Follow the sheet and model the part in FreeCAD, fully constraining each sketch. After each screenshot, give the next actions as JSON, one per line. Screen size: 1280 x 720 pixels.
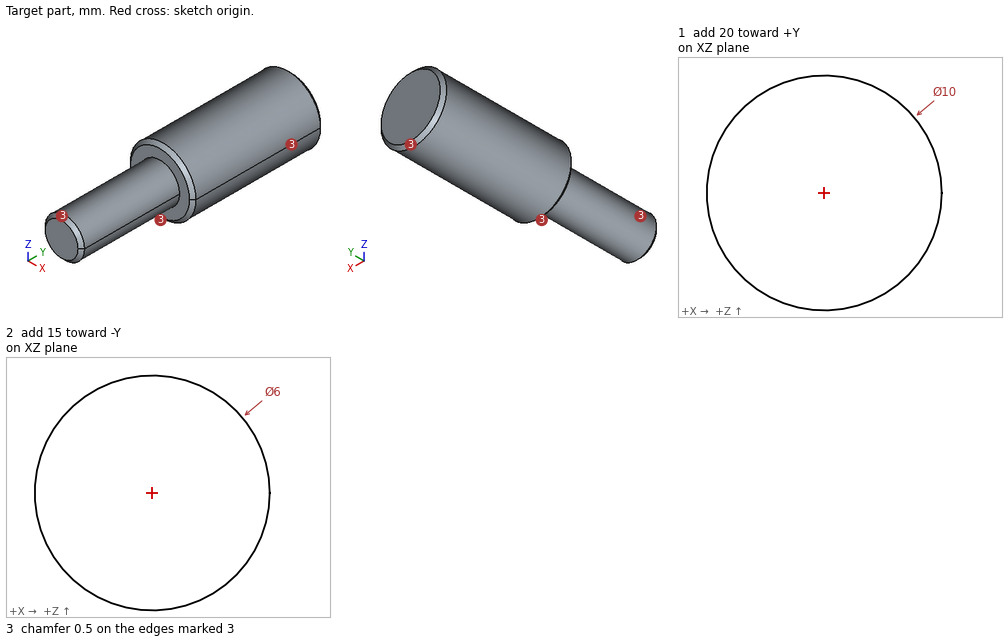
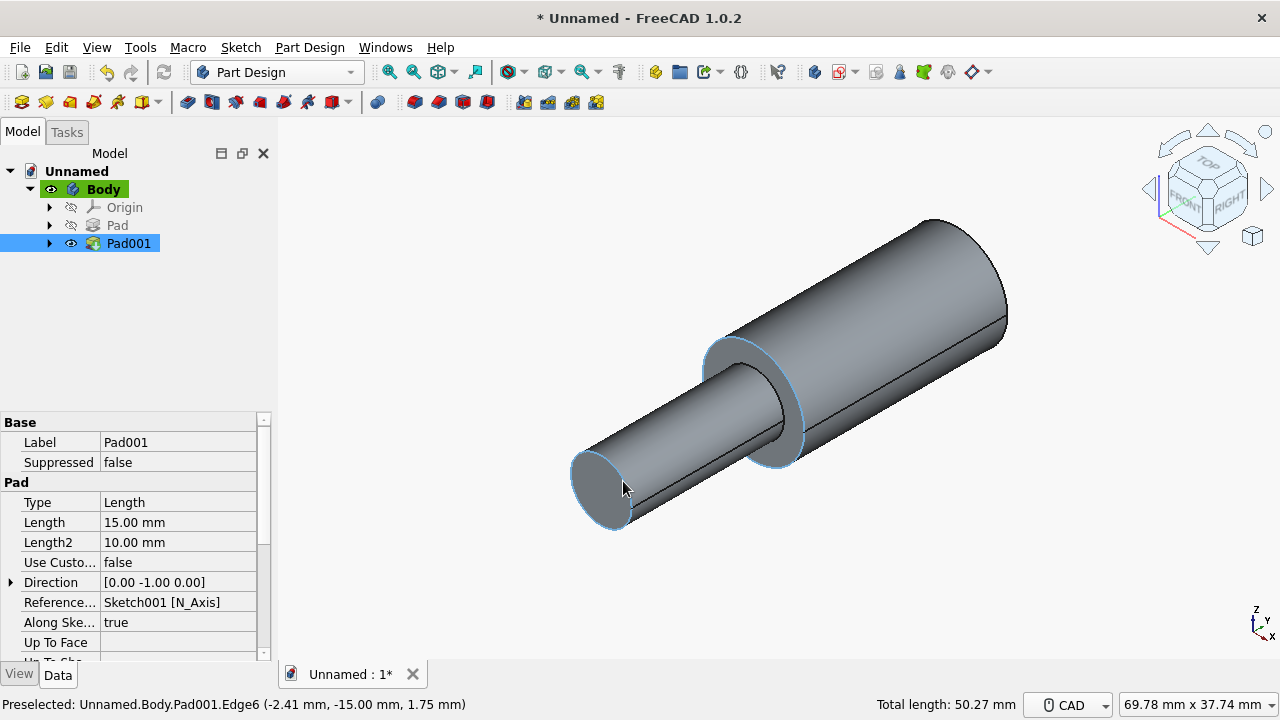
{"action": "key", "text": "2"}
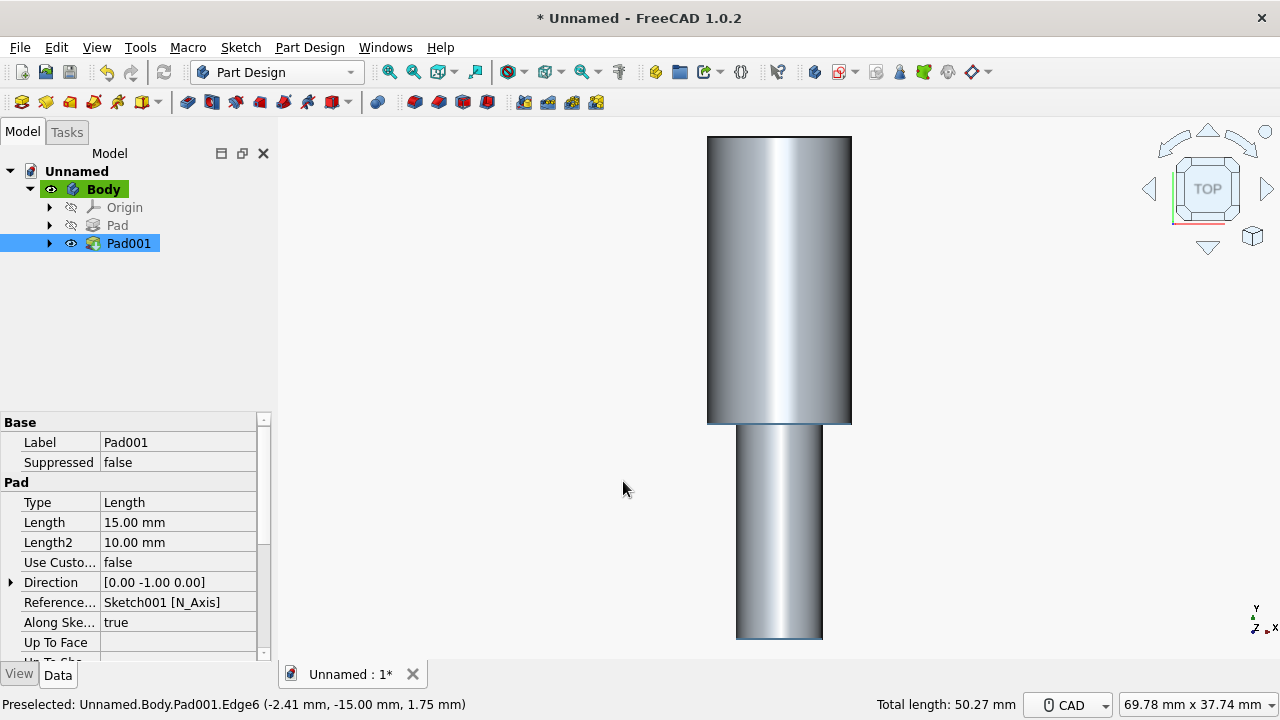
{"action": "key", "text": "1"}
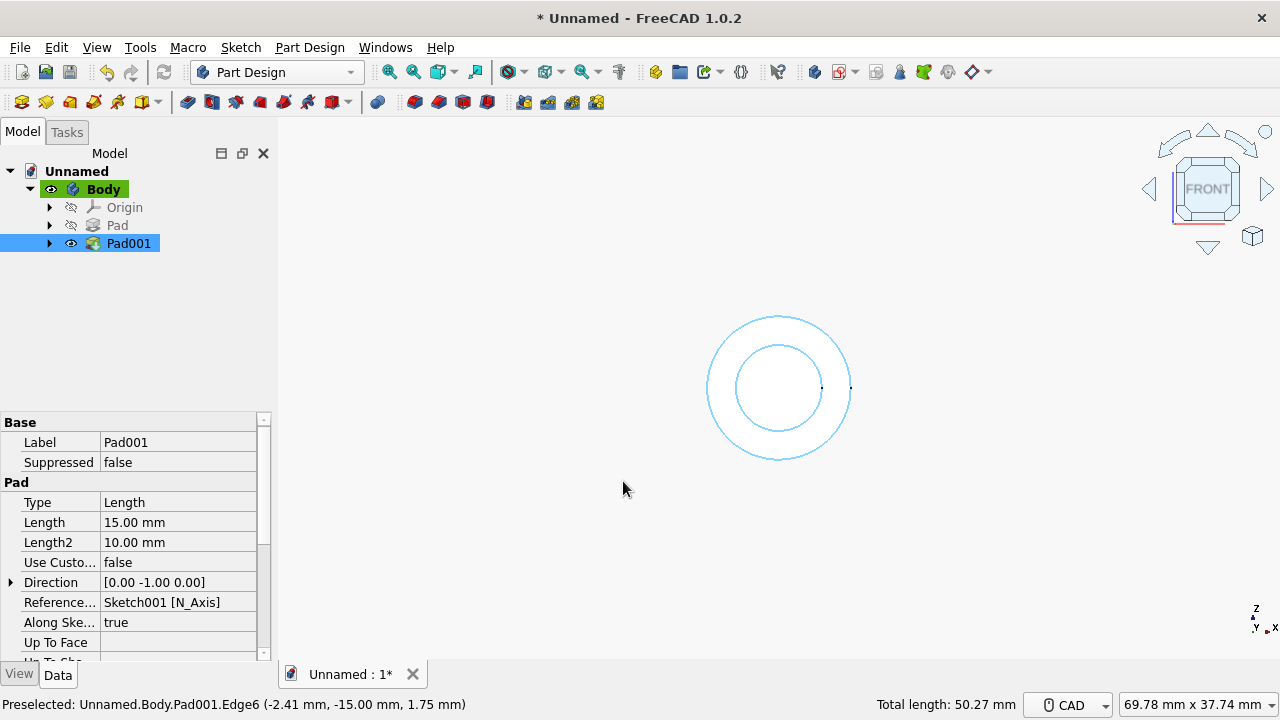
{"action": "left_click", "coordinate": [390, 72]}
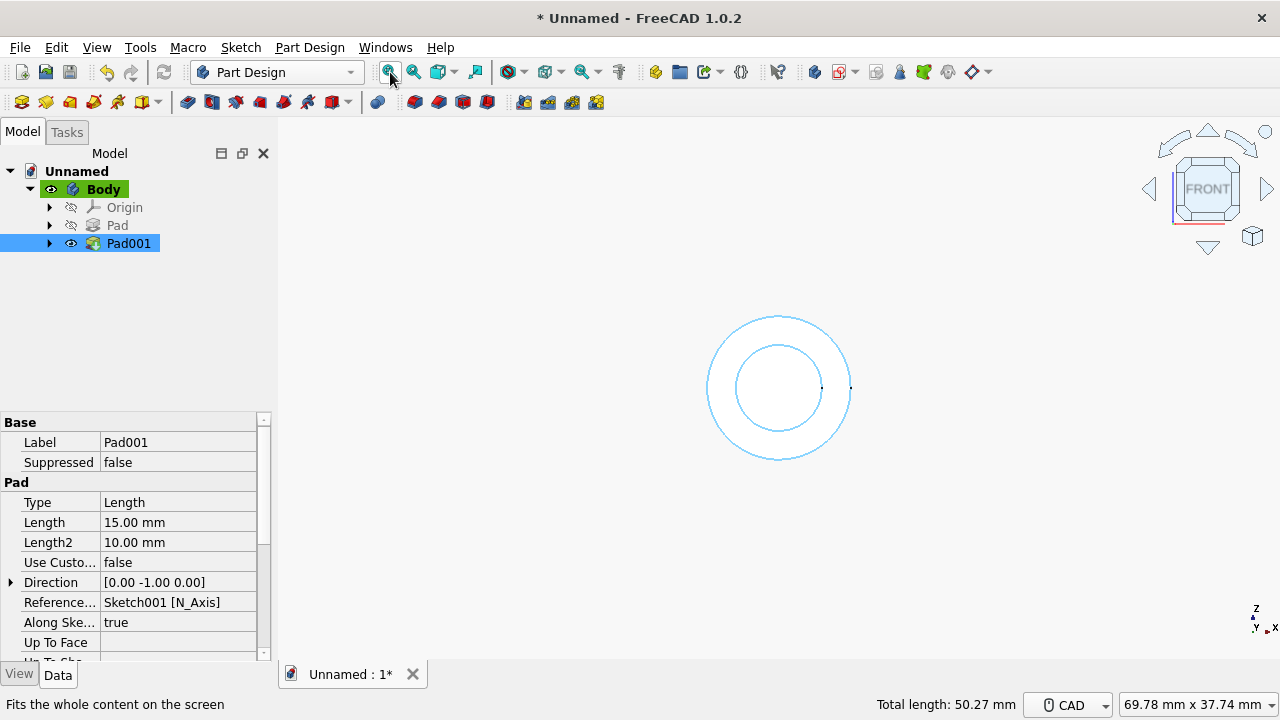
{"action": "key", "text": "3"}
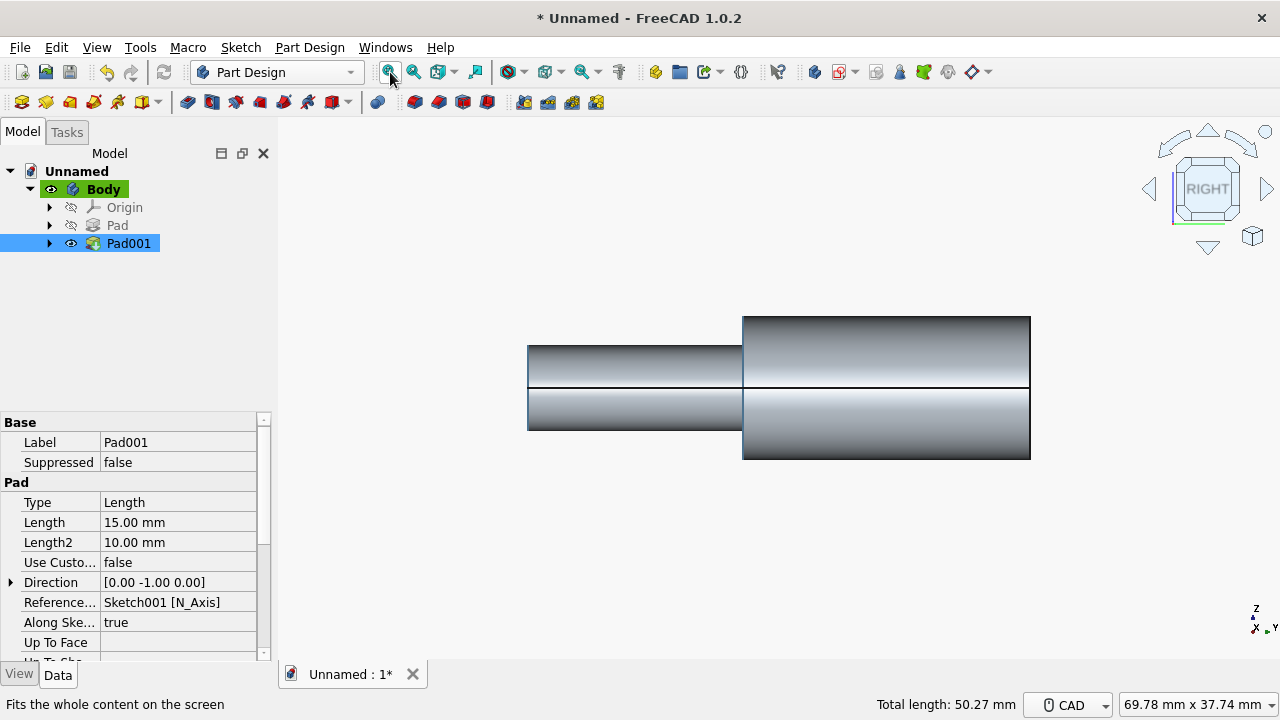
{"action": "left_click", "coordinate": [1030, 345], "text": "ctrl"}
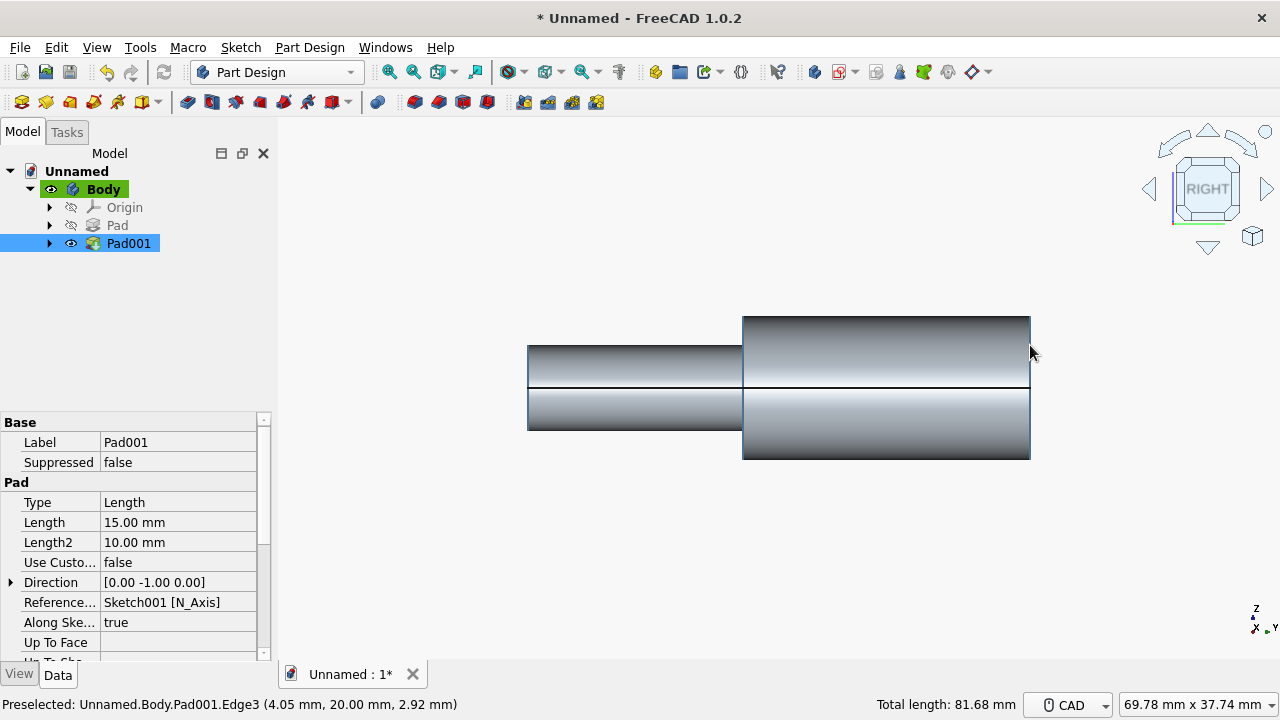
{"action": "left_click", "coordinate": [440, 102]}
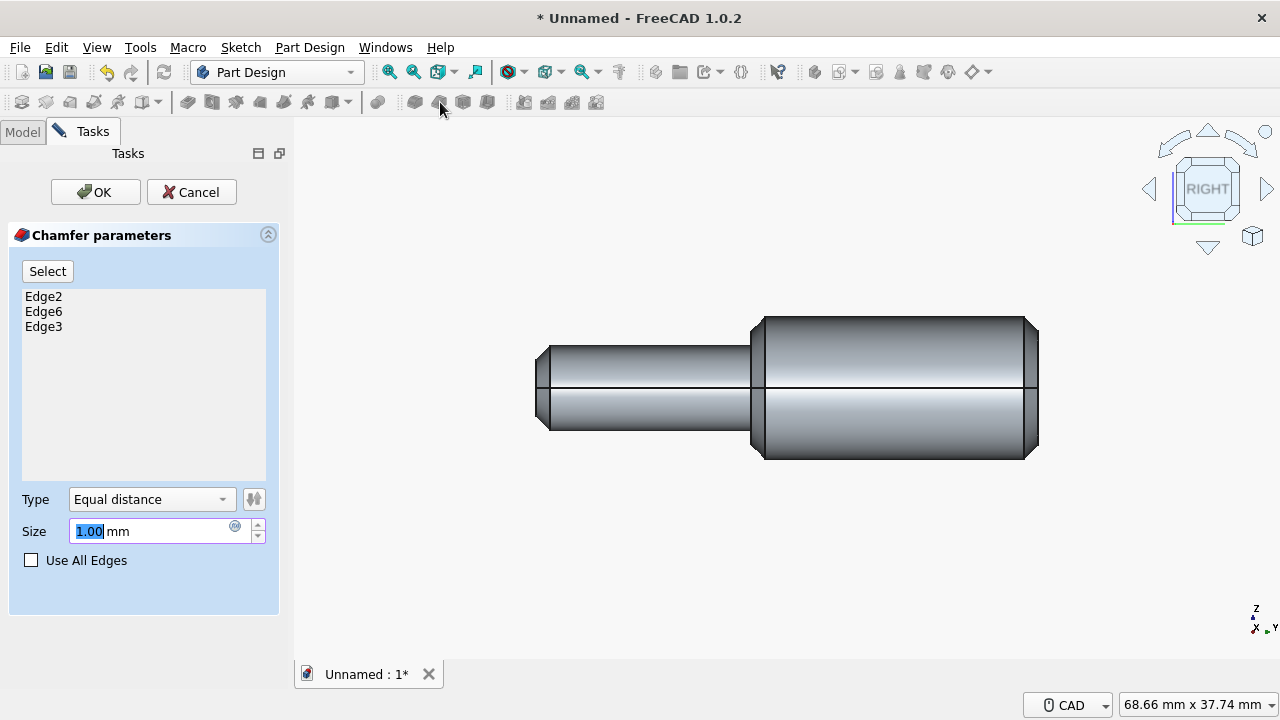
{"action": "type", "text": "0.5"}
{"action": "key", "text": "Tab"}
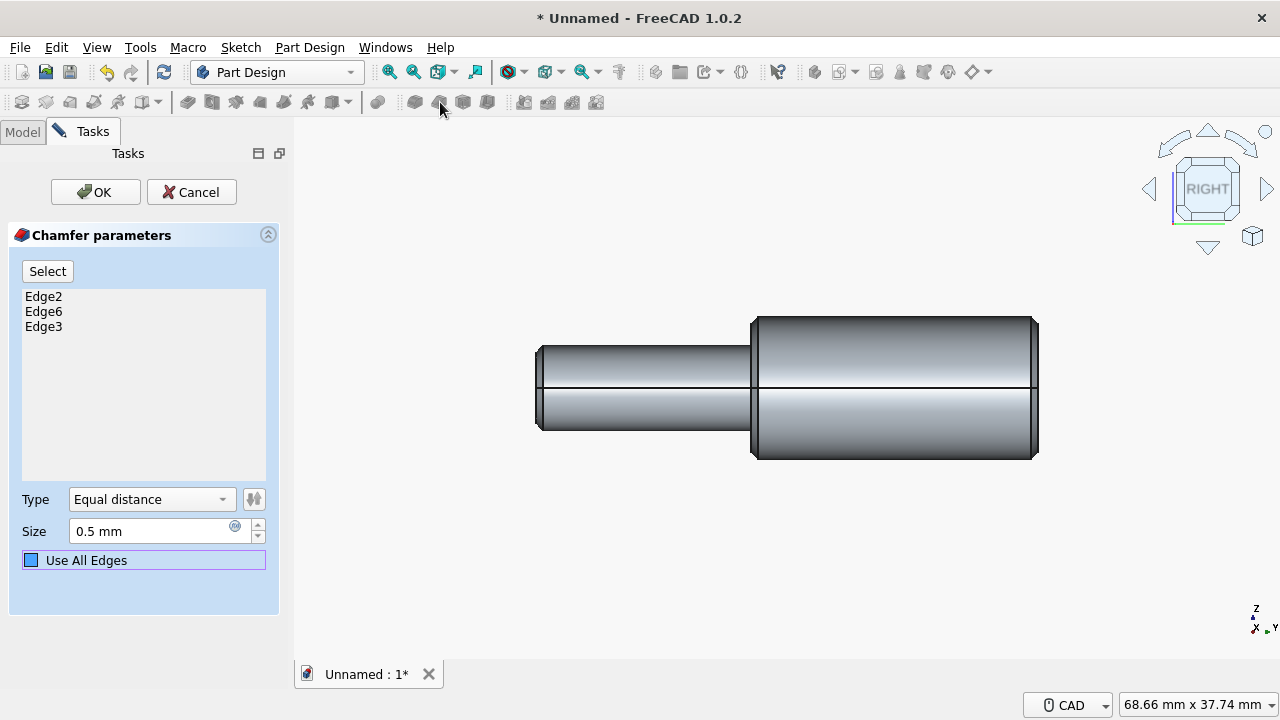
{"action": "left_click", "coordinate": [96, 192]}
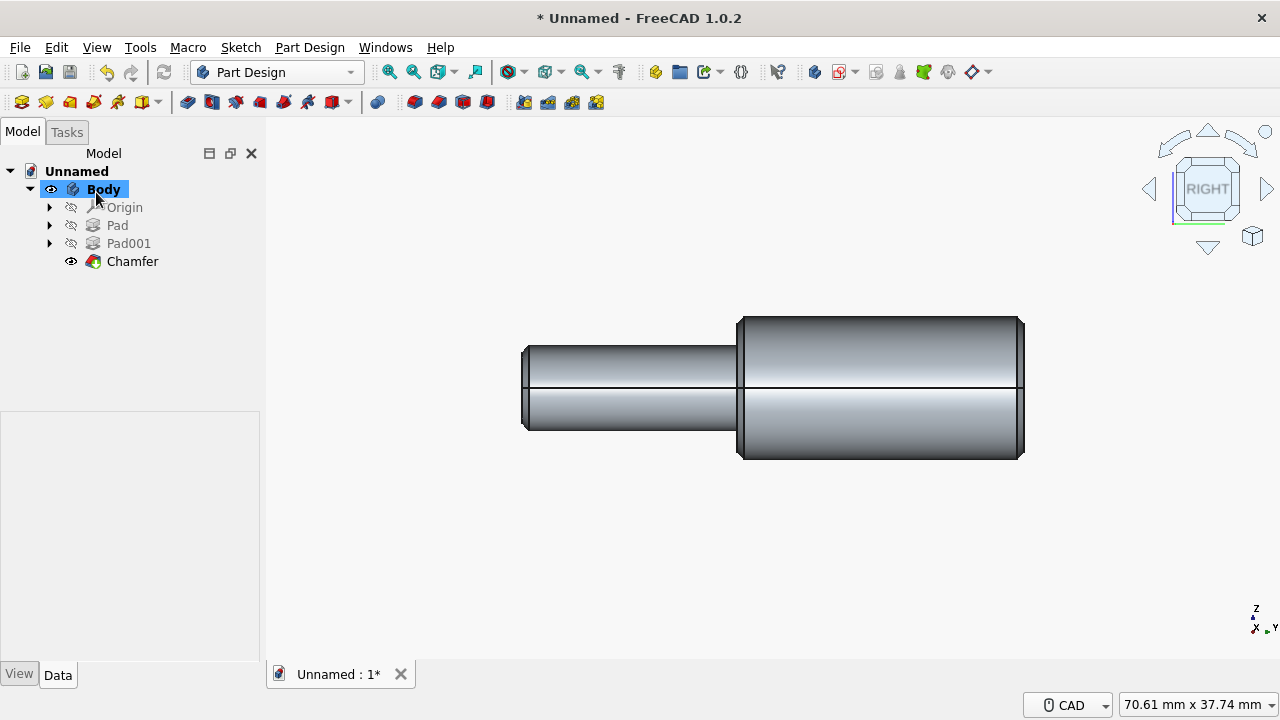
{"action": "key", "text": "0"}